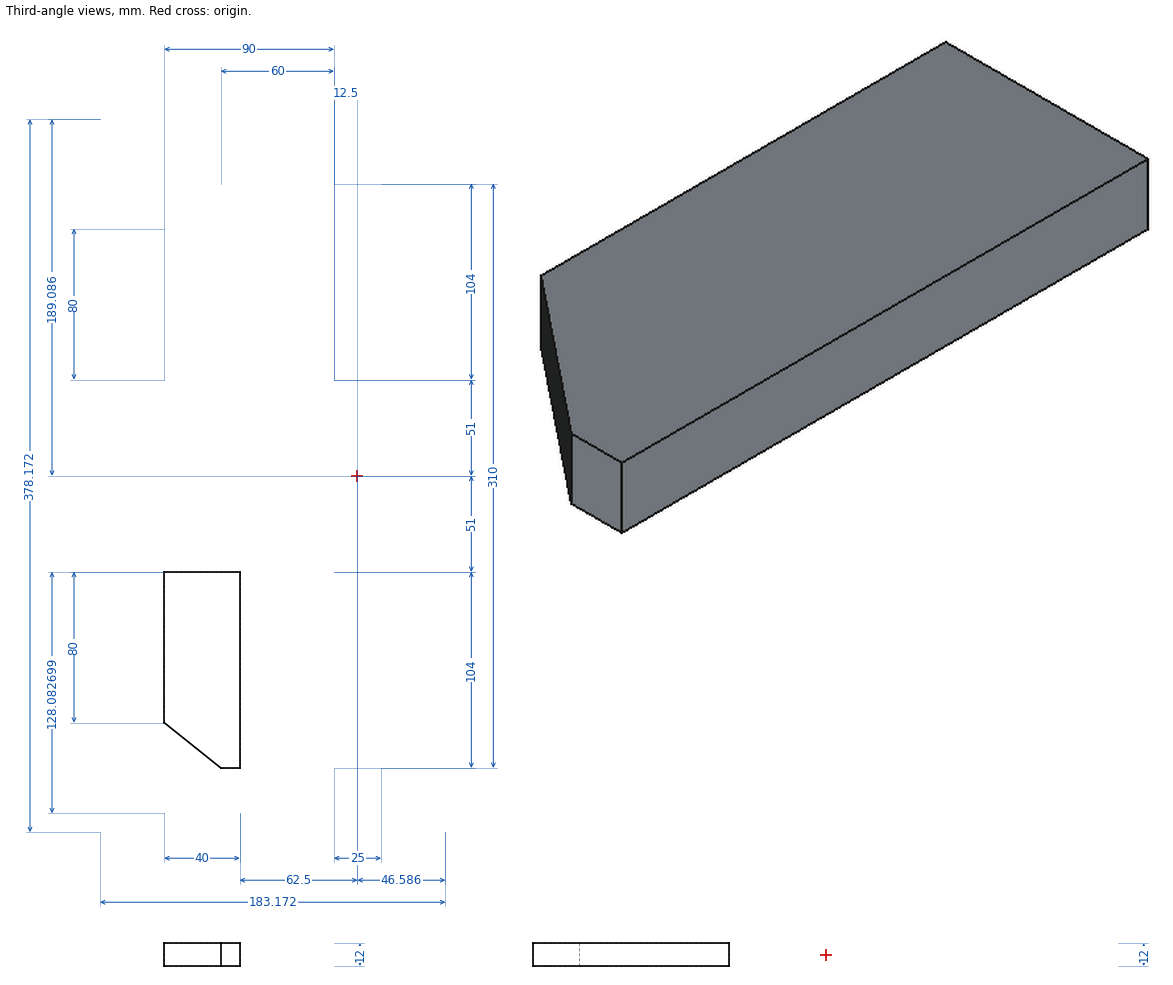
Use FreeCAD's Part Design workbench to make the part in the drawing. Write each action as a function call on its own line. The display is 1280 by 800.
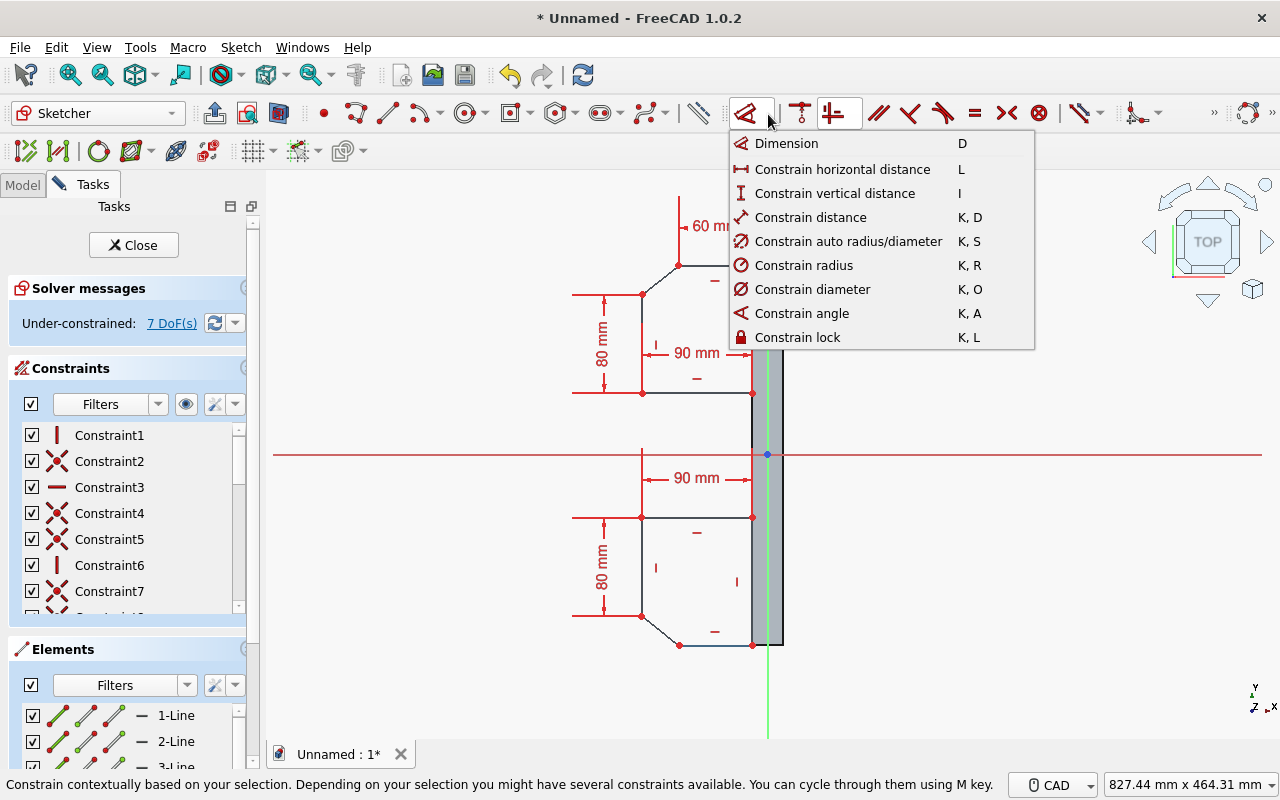
click(882, 169)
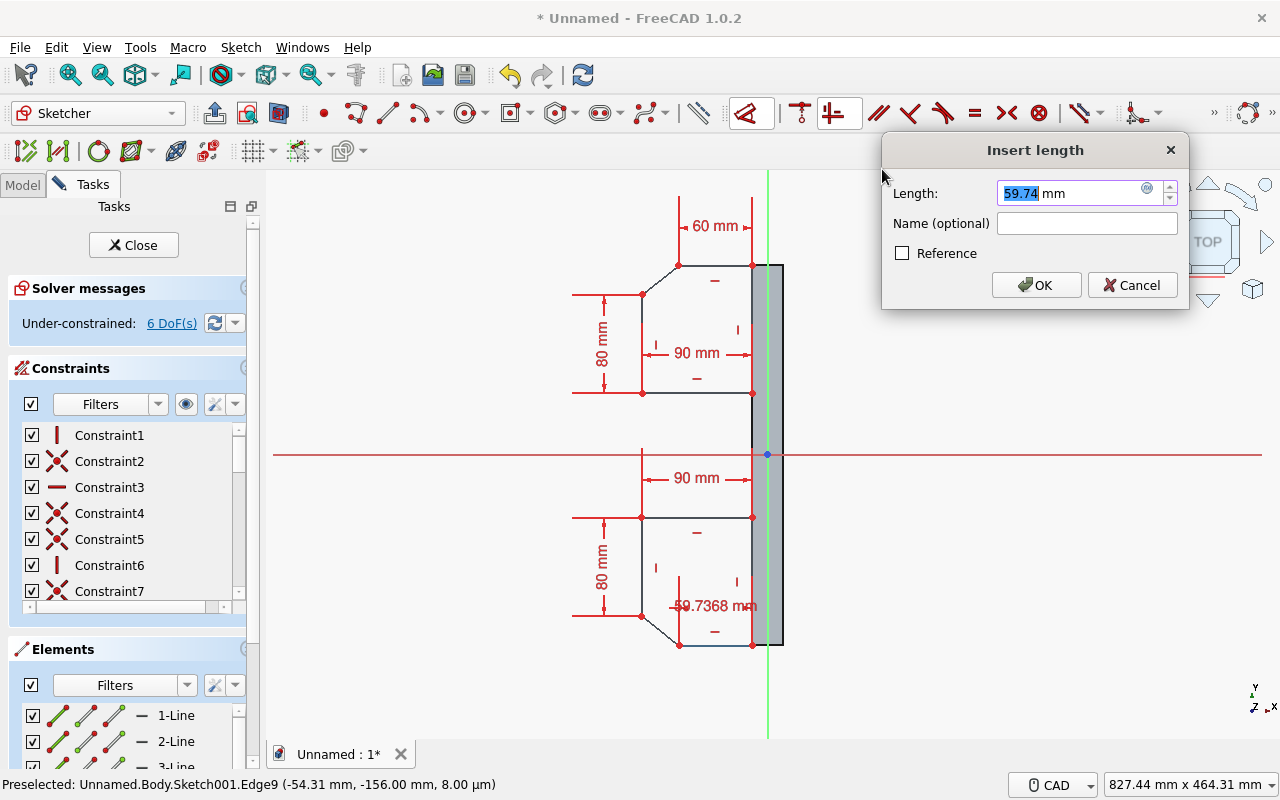
text(60)
key(Return)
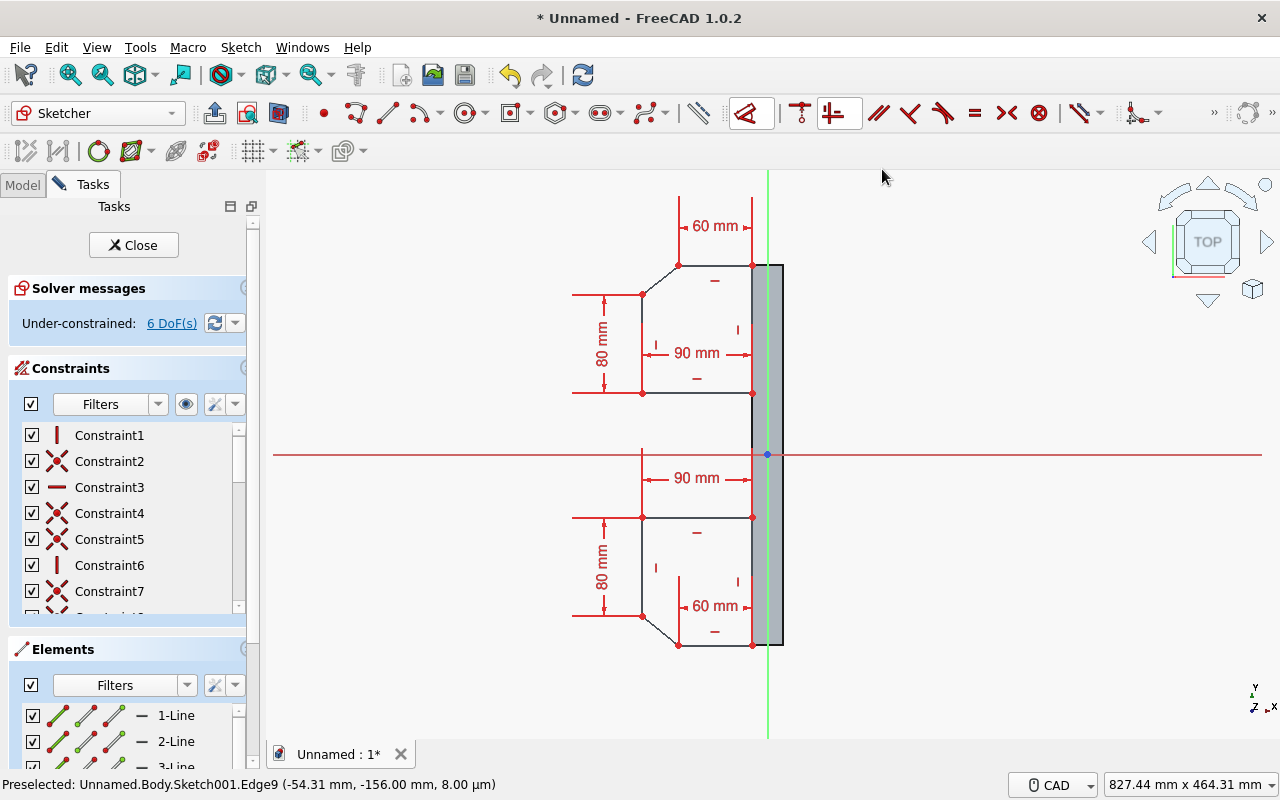
click(752, 355)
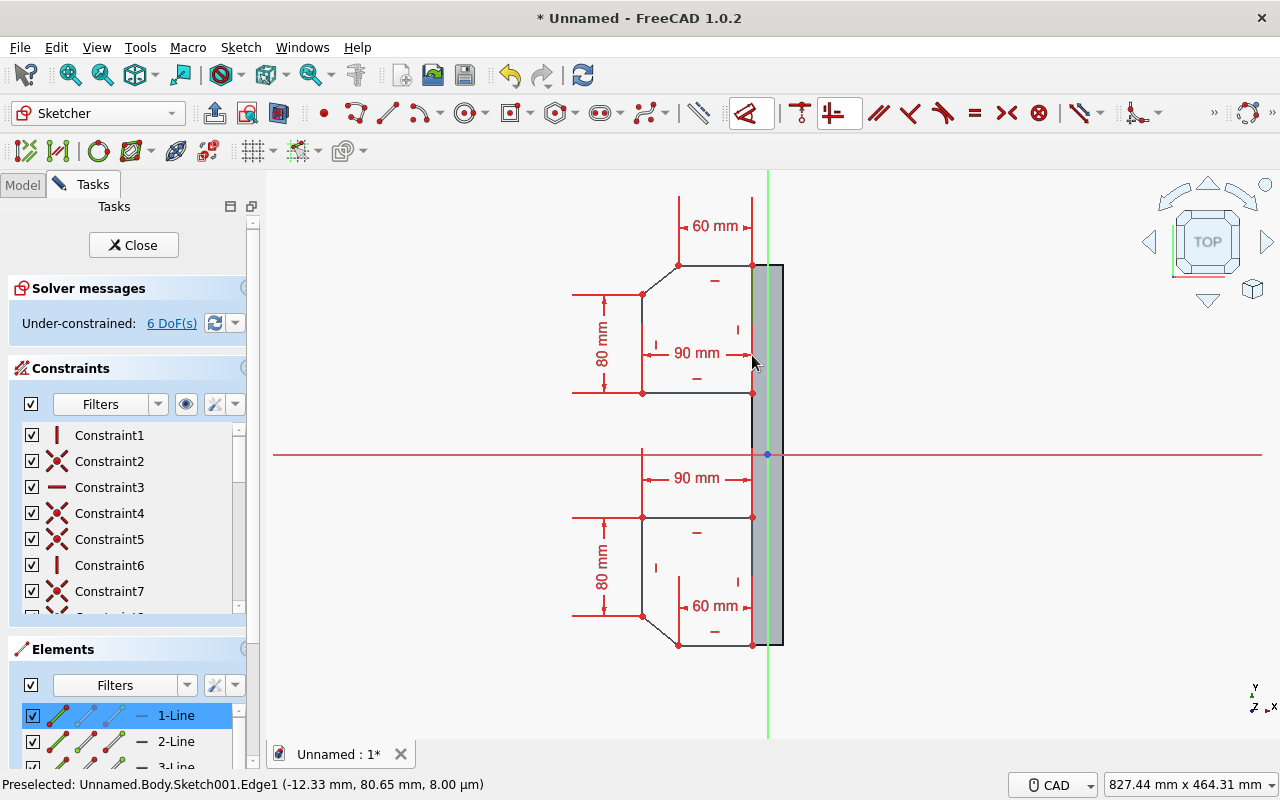
click(768, 114)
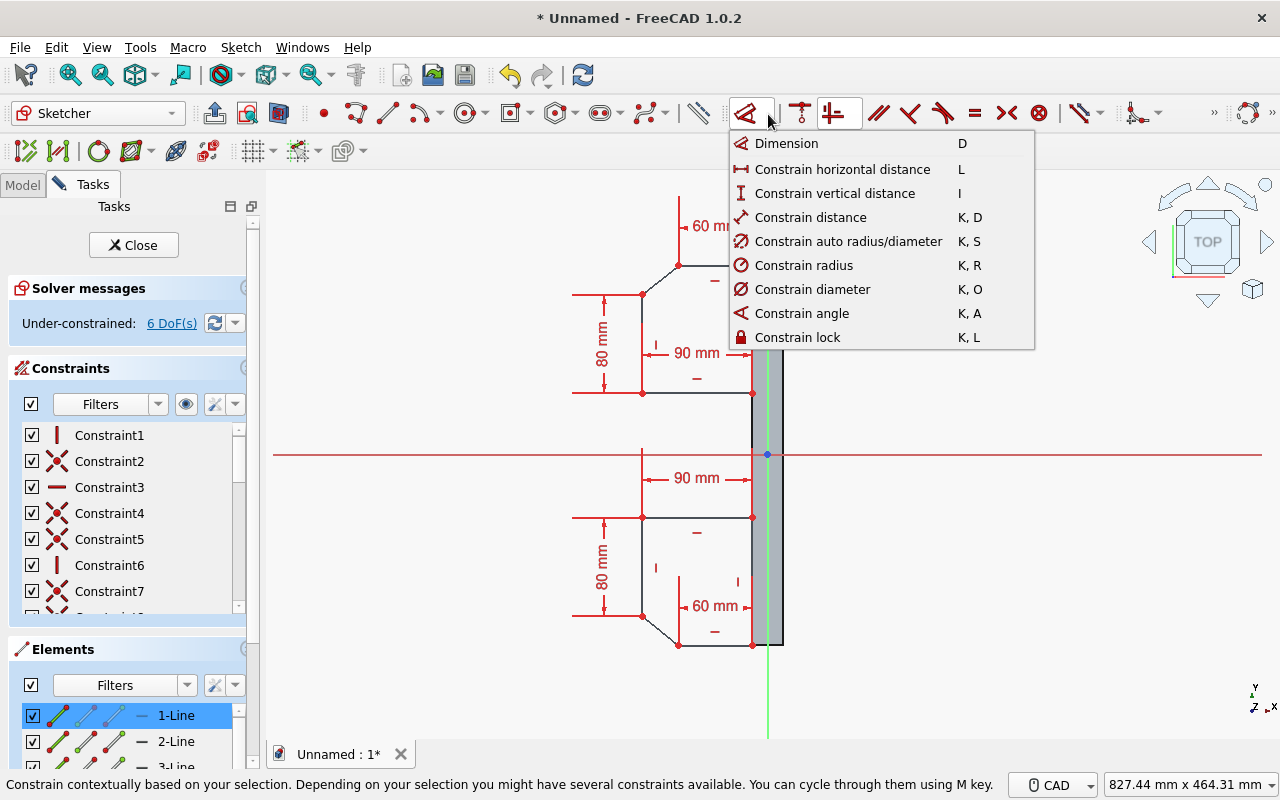
click(882, 193)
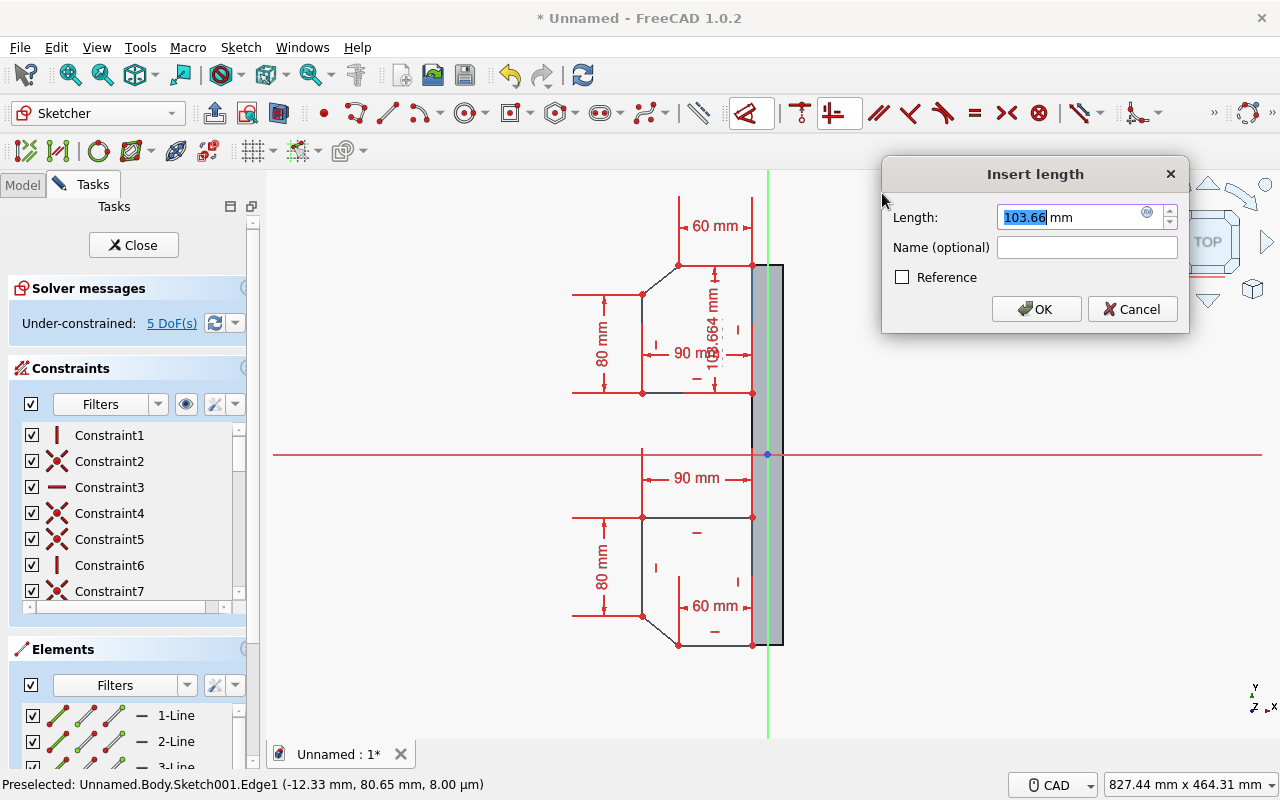
text(104)
key(Return)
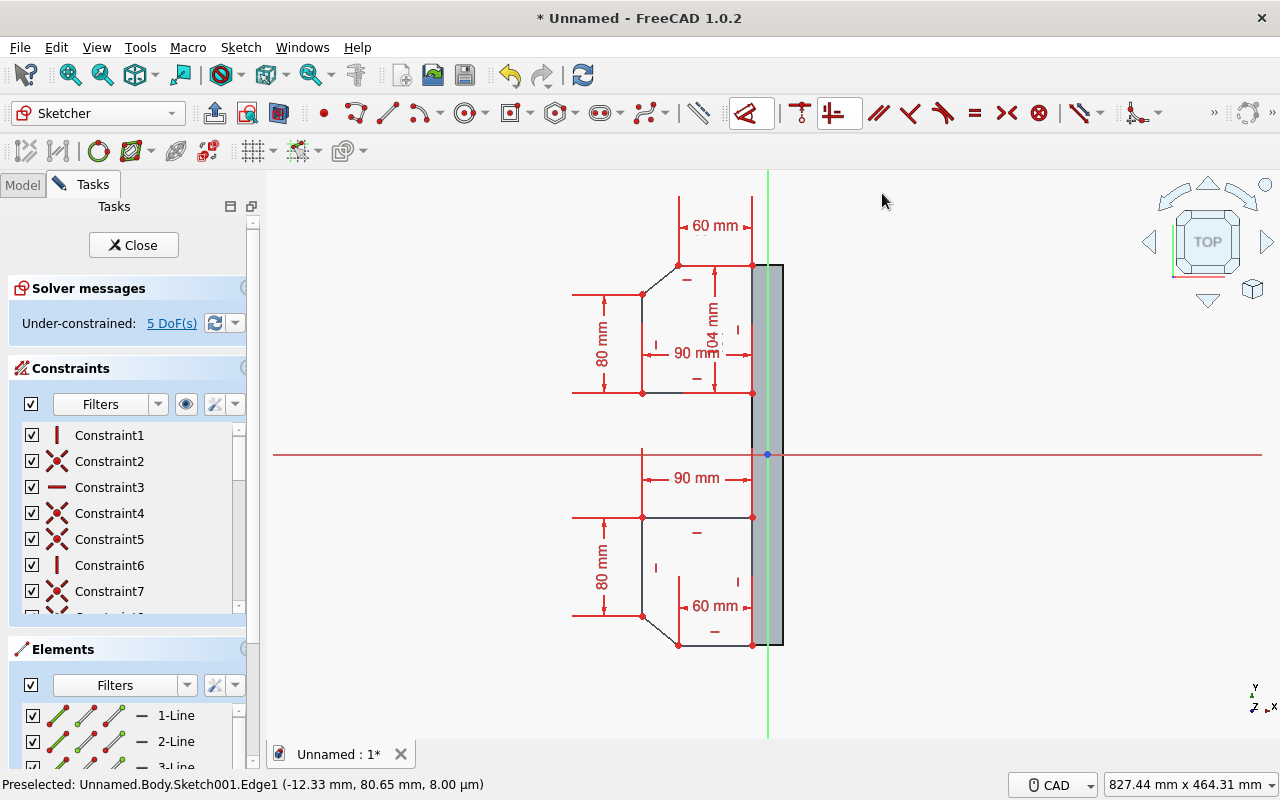
click(752, 608)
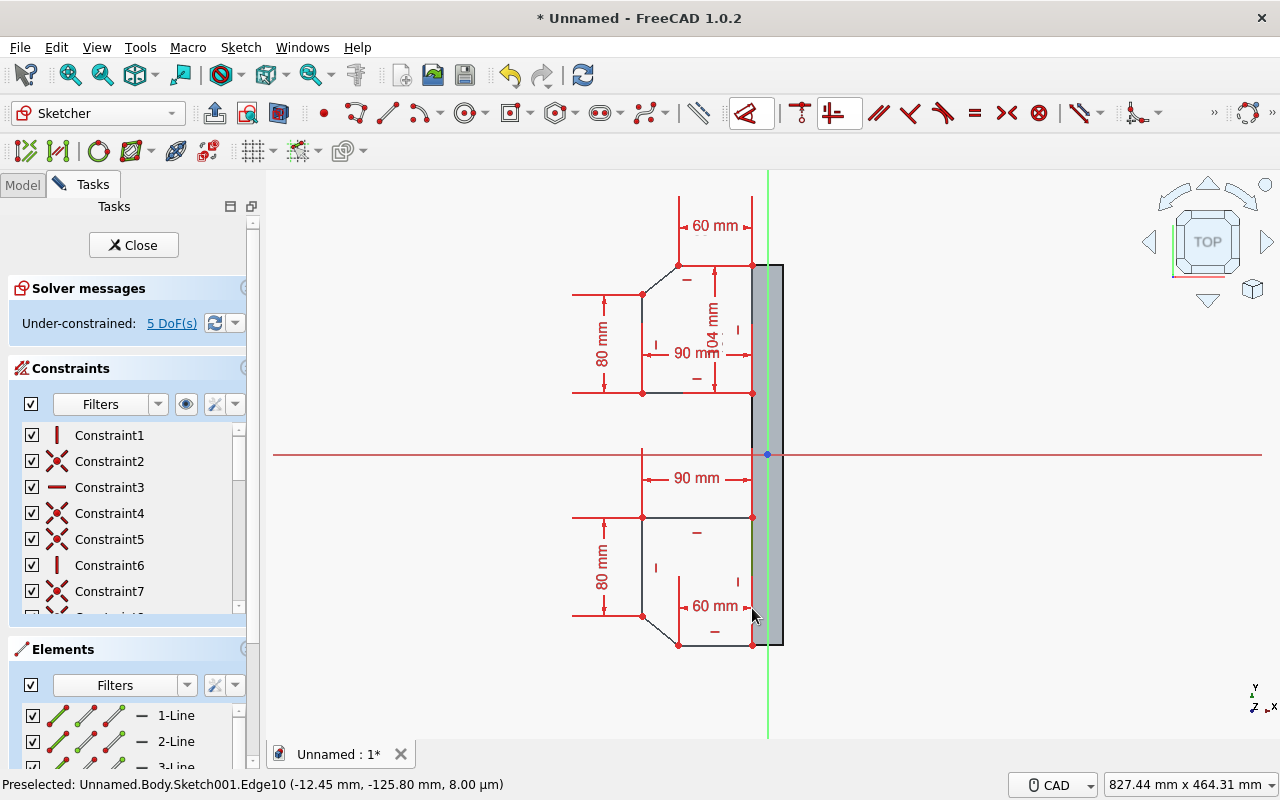
click(768, 114)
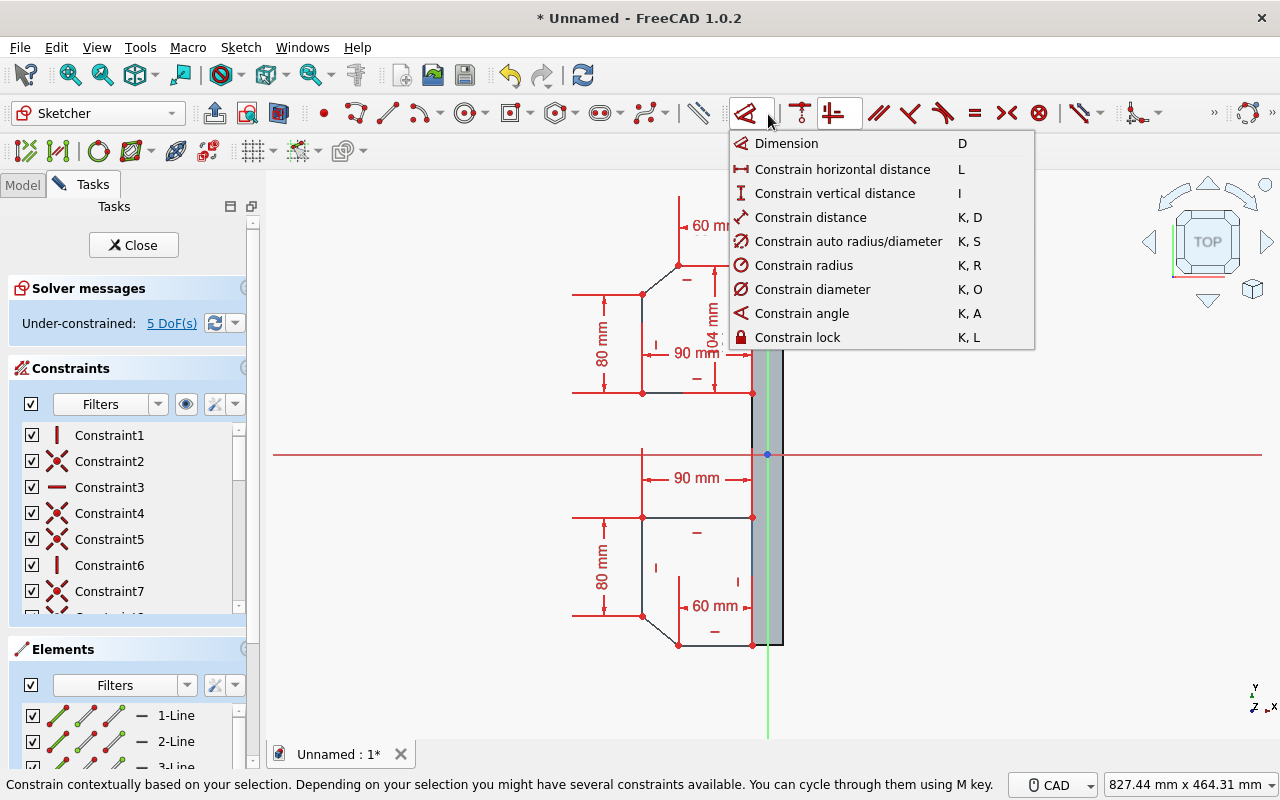
click(882, 193)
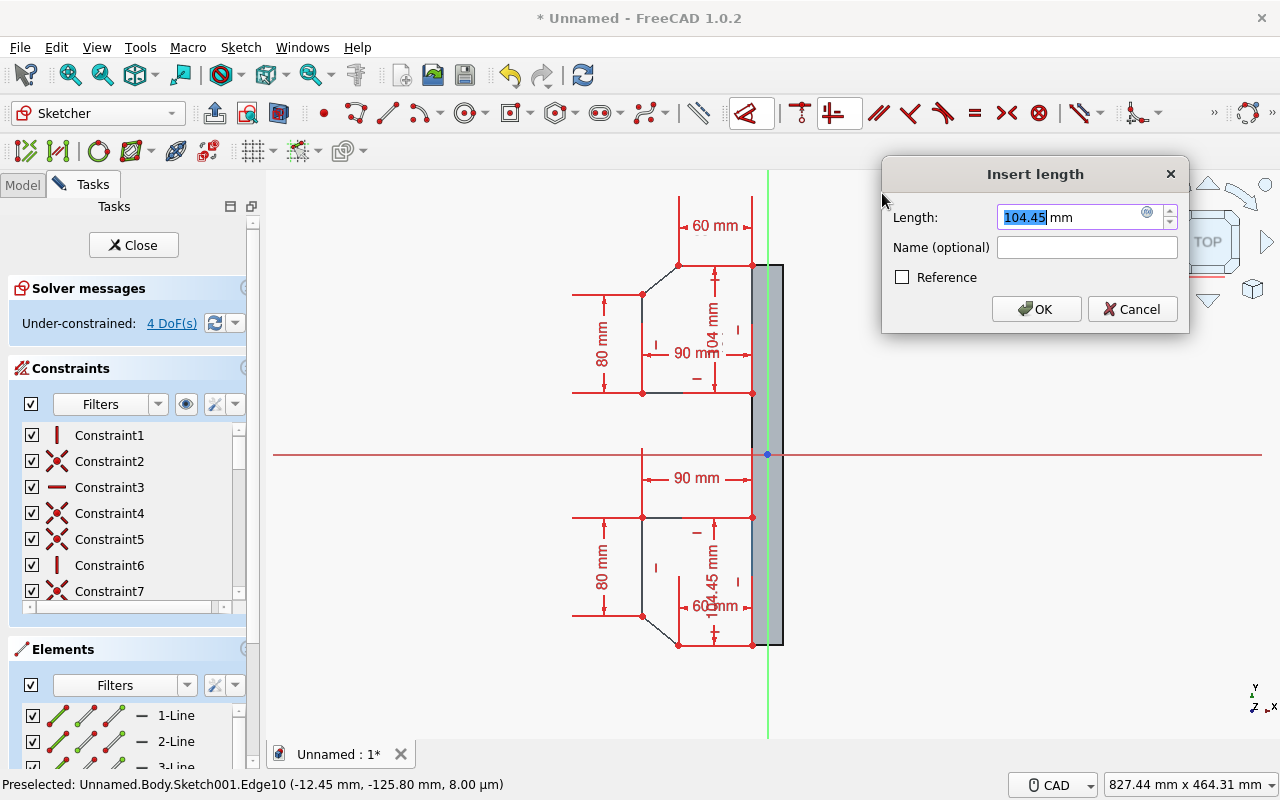
text(104)
key(Return)